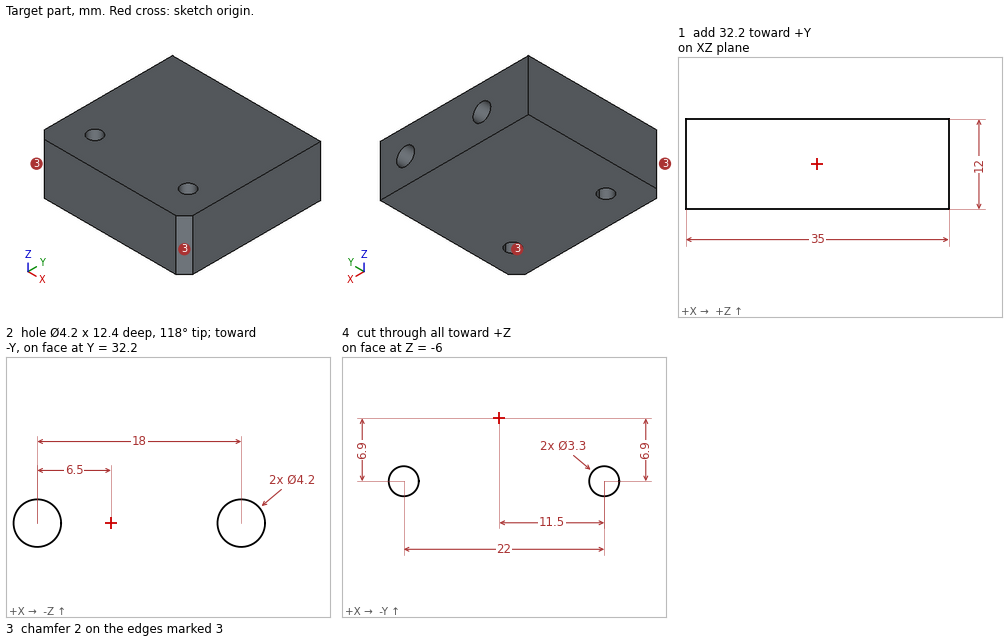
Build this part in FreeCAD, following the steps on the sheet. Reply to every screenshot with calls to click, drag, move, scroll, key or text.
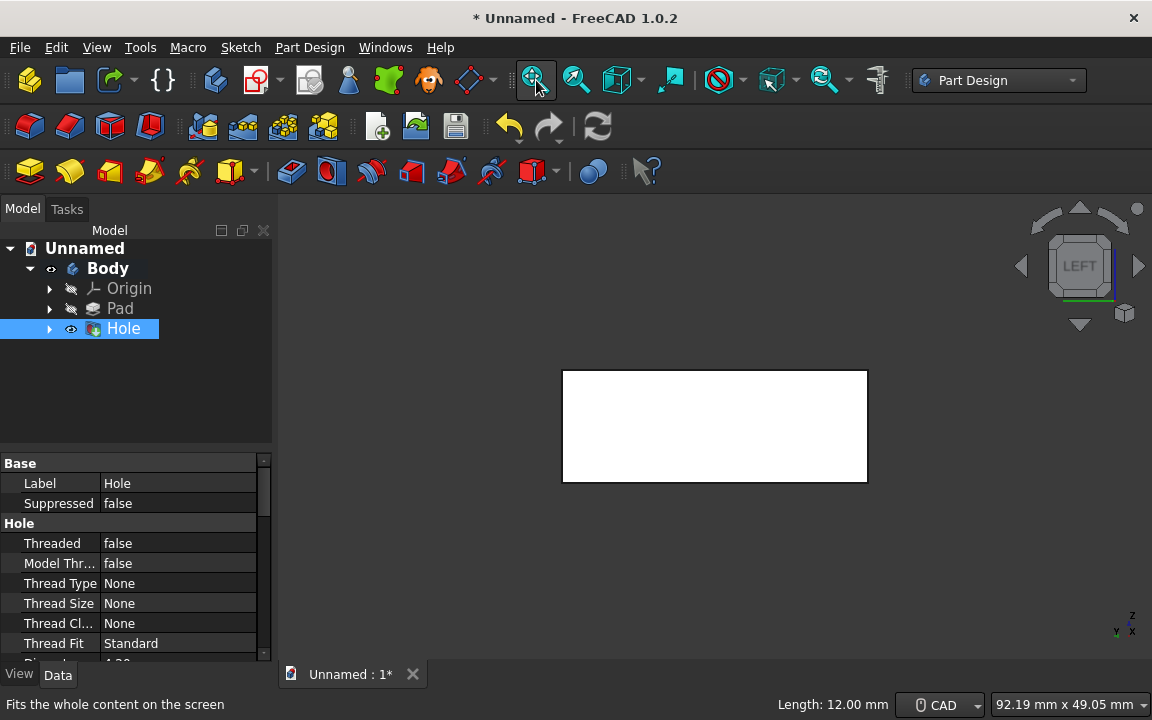
click(536, 80)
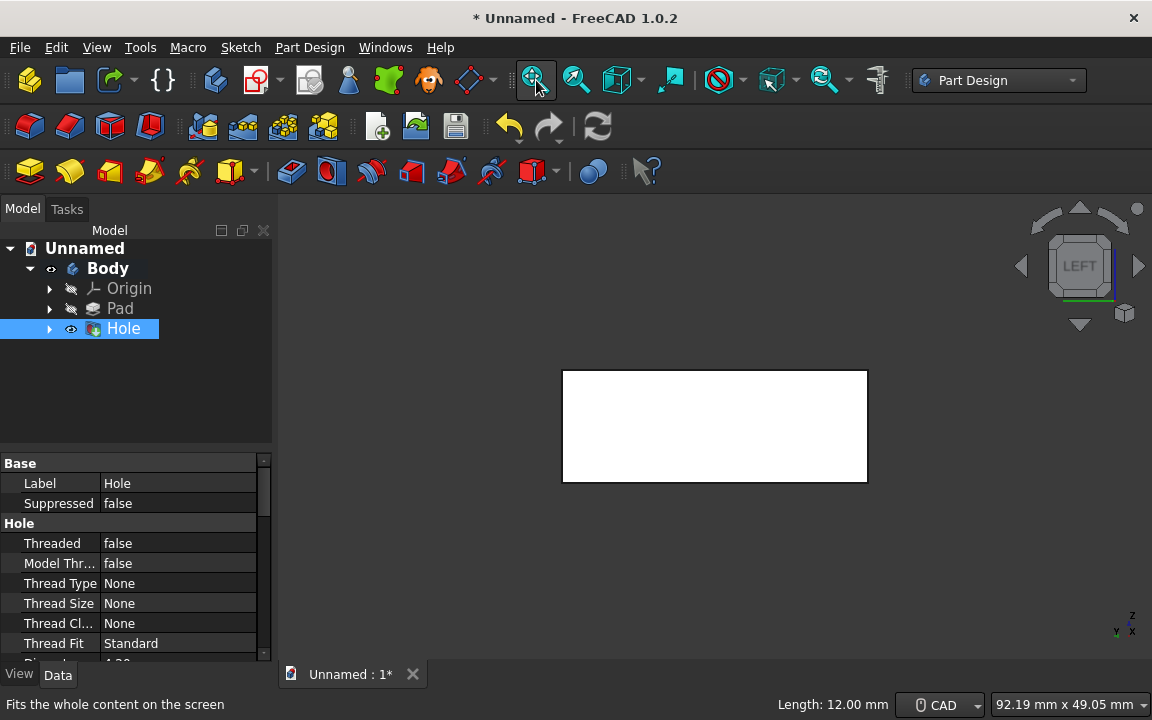
click(868, 426, ctrl)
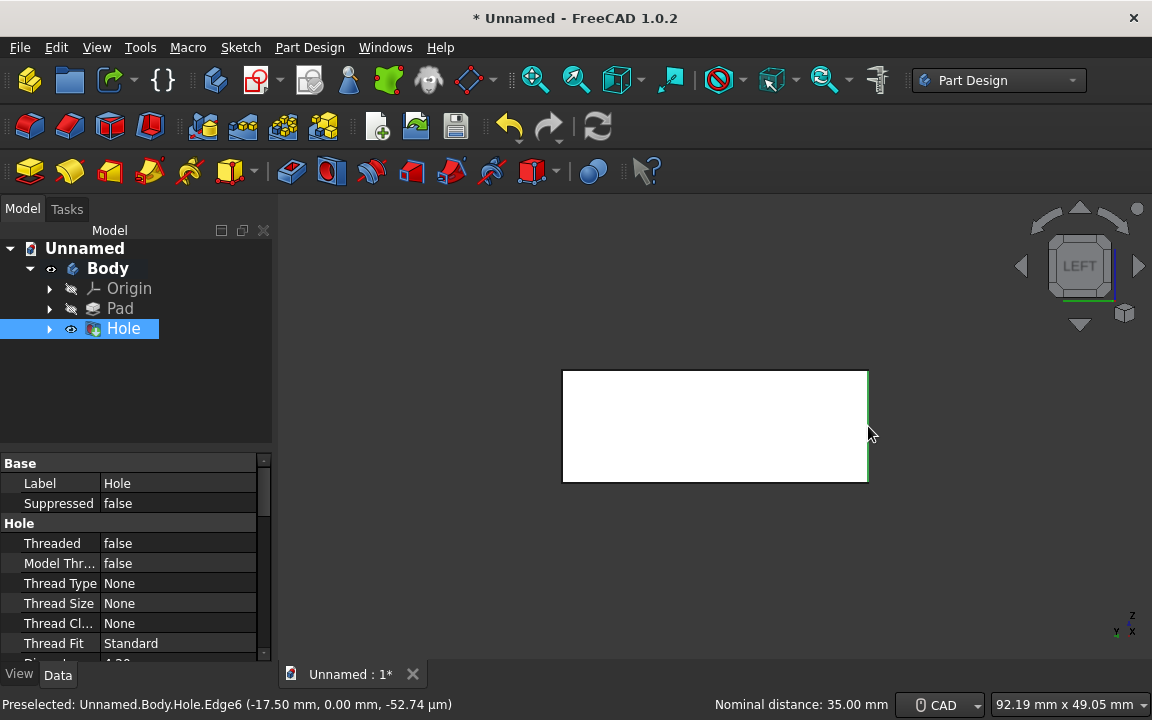
click(70, 126)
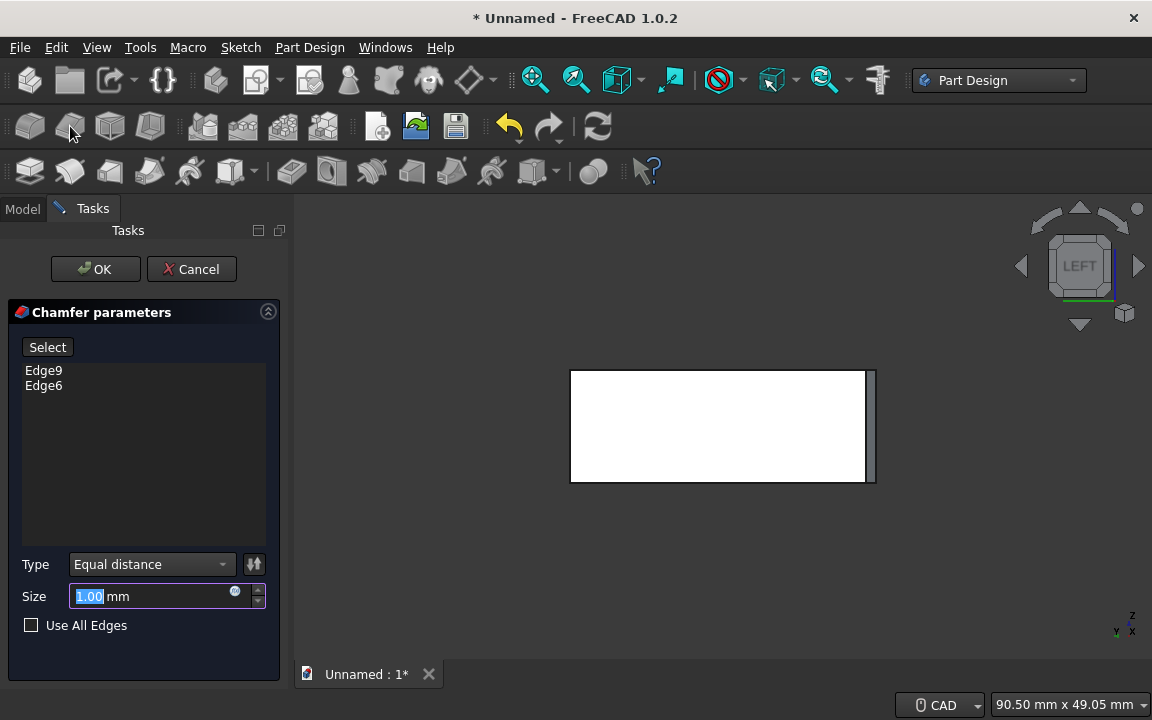
text(2)
key(Tab)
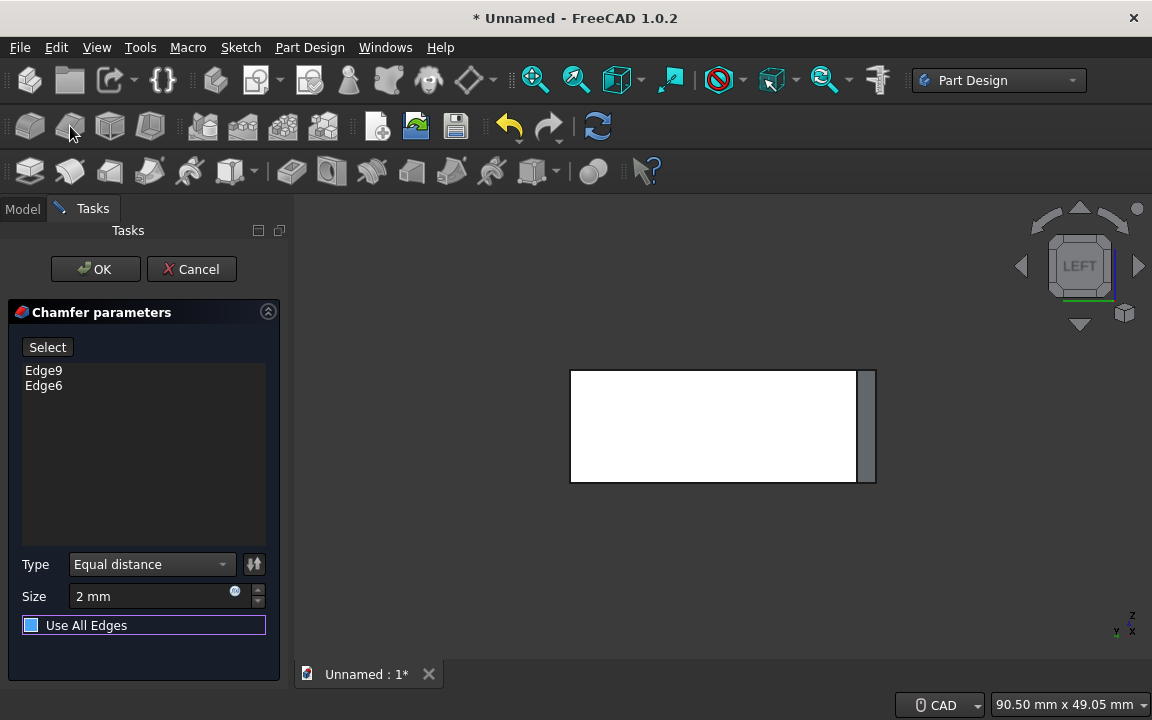
click(96, 269)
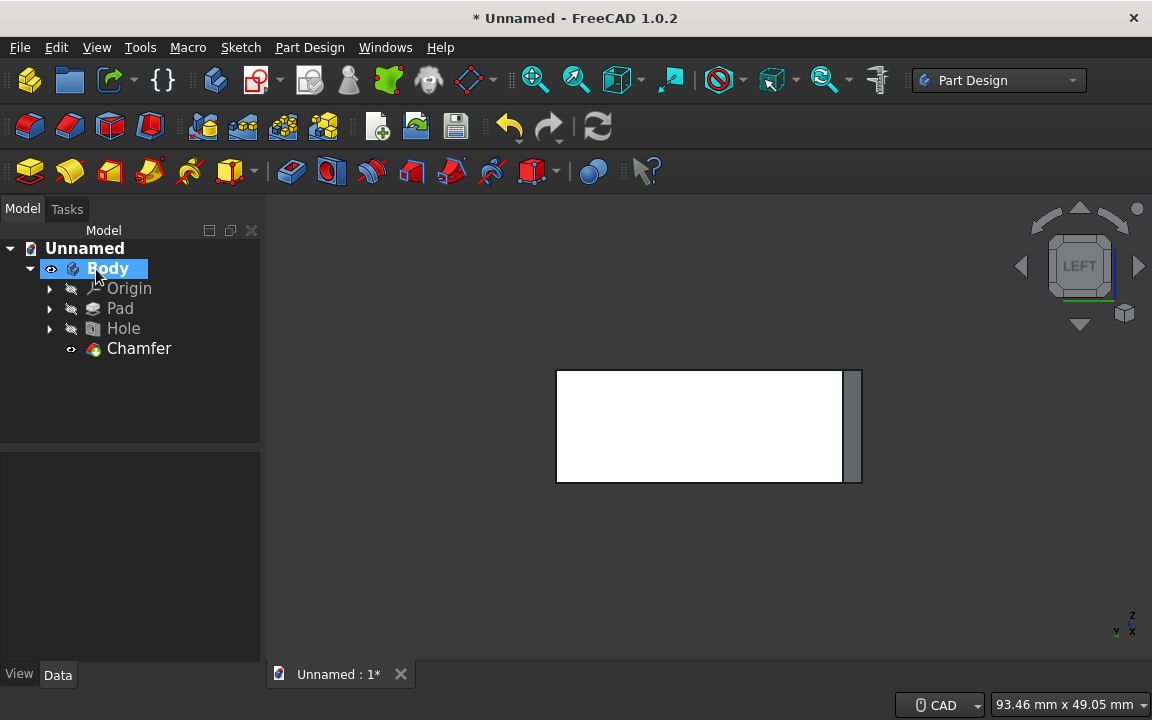
key(v)
key(f)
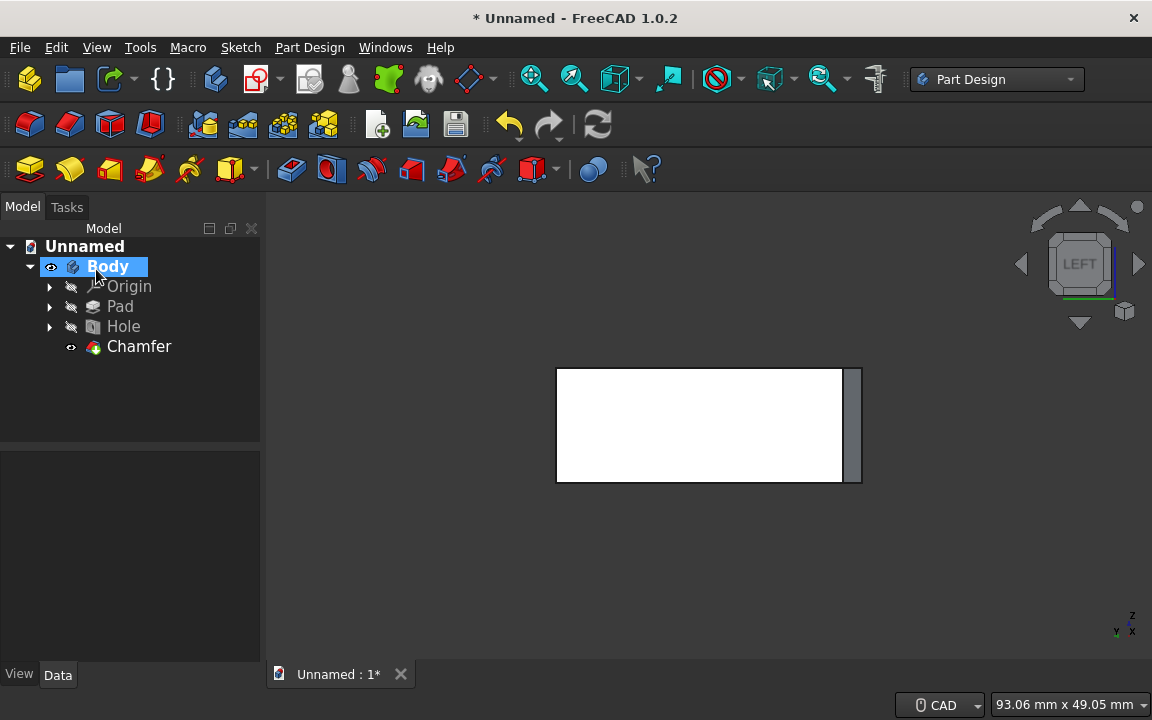
key(5)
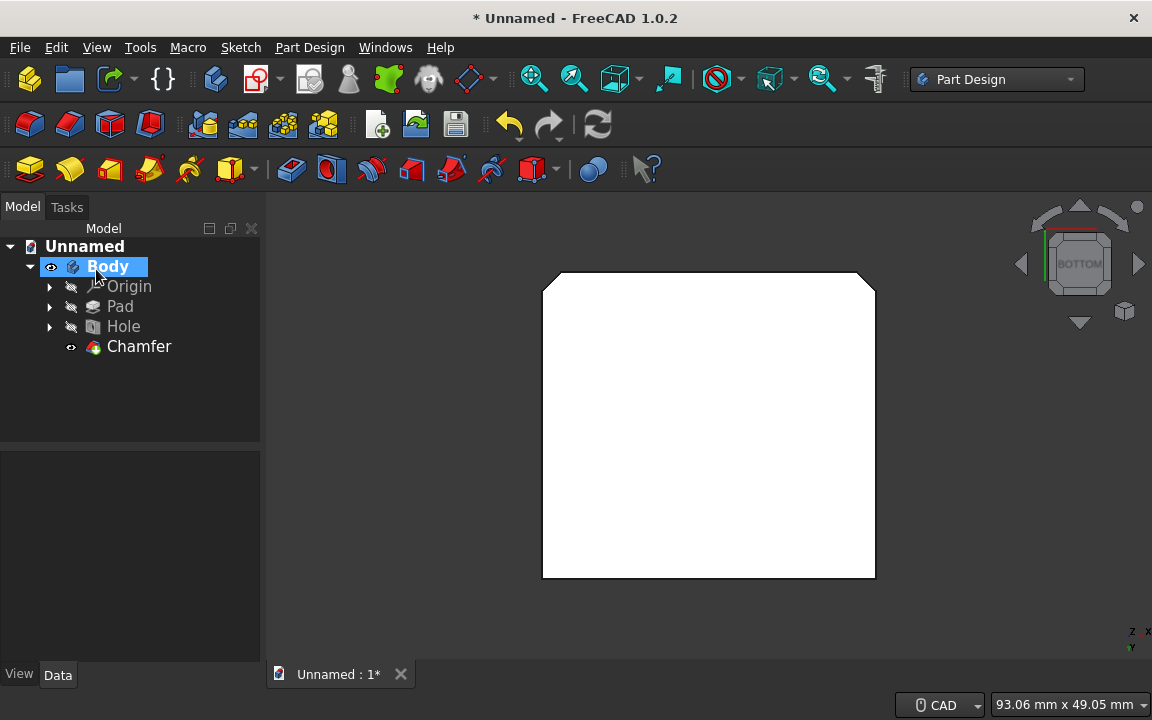
click(709, 424)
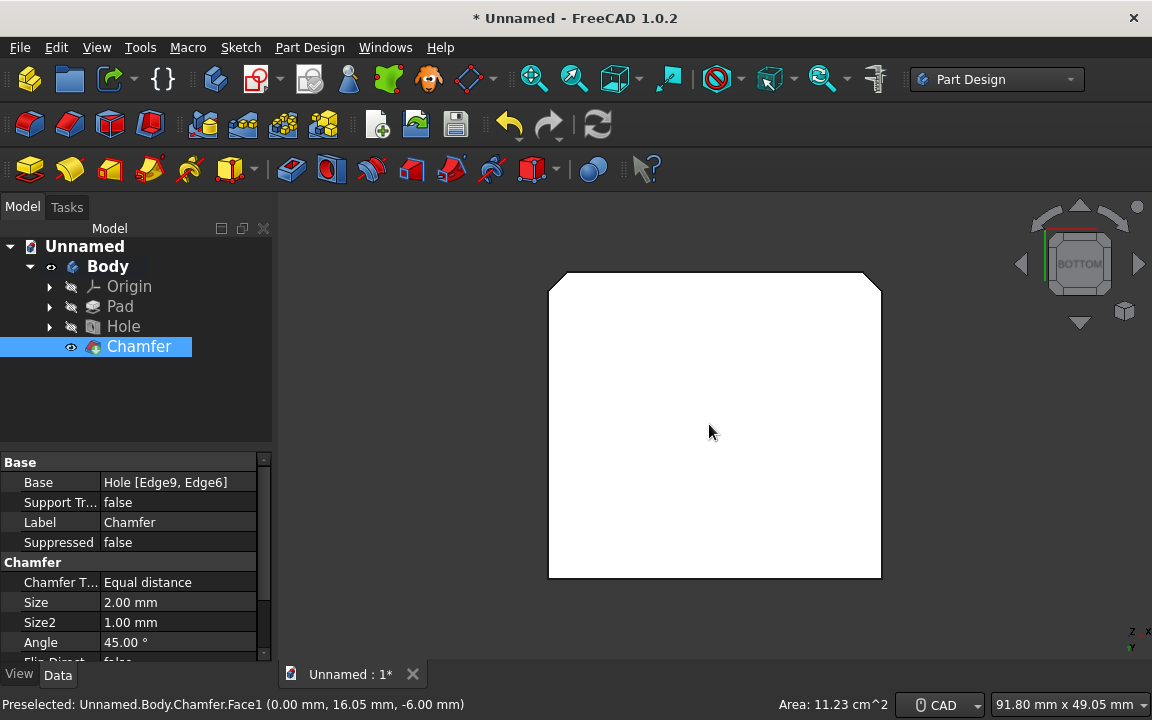
click(256, 80)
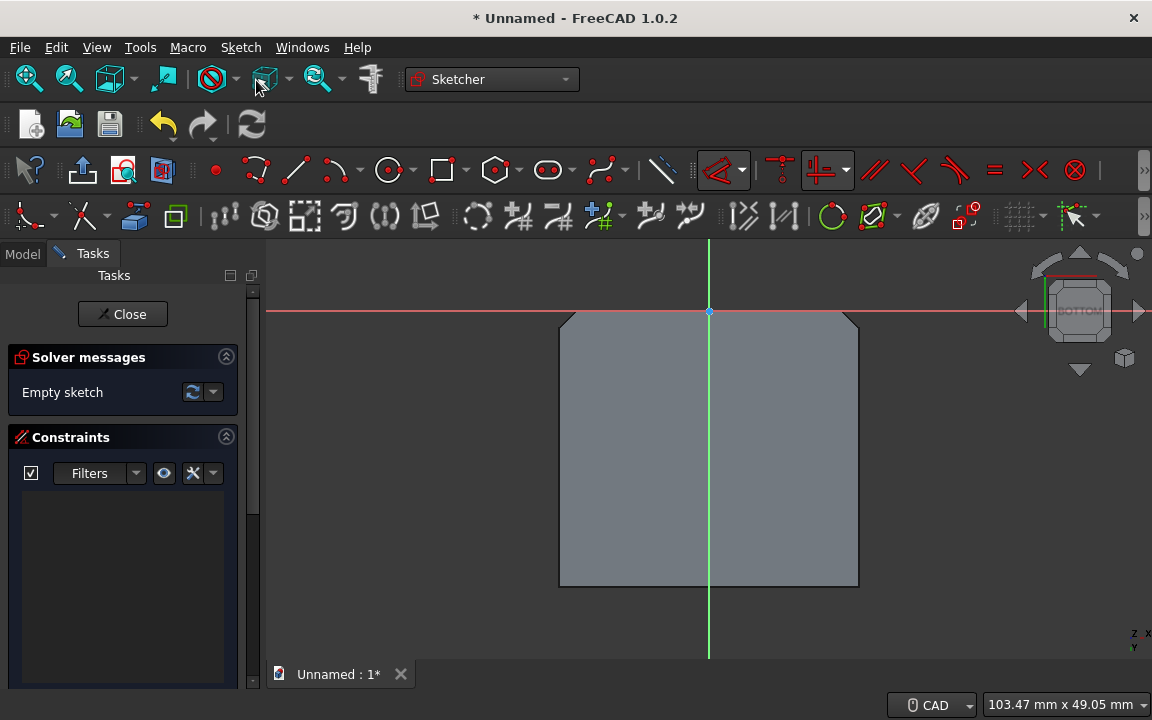
scroll(773, 267, up, 4)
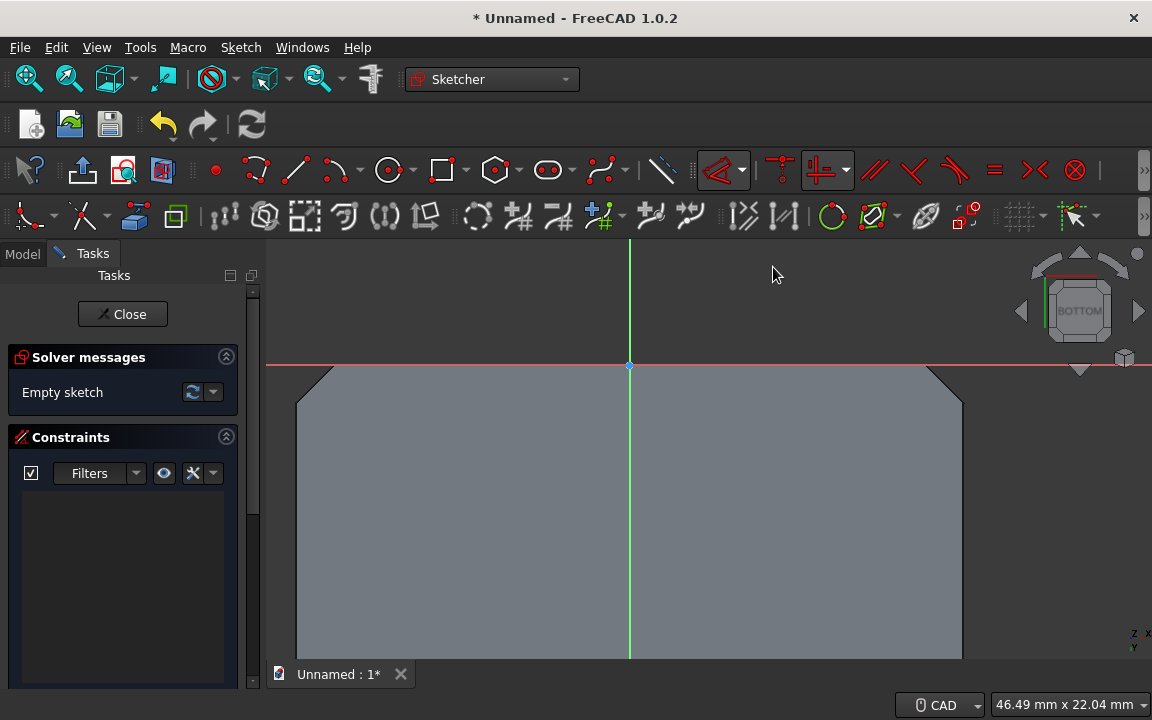
key(g)
key(c)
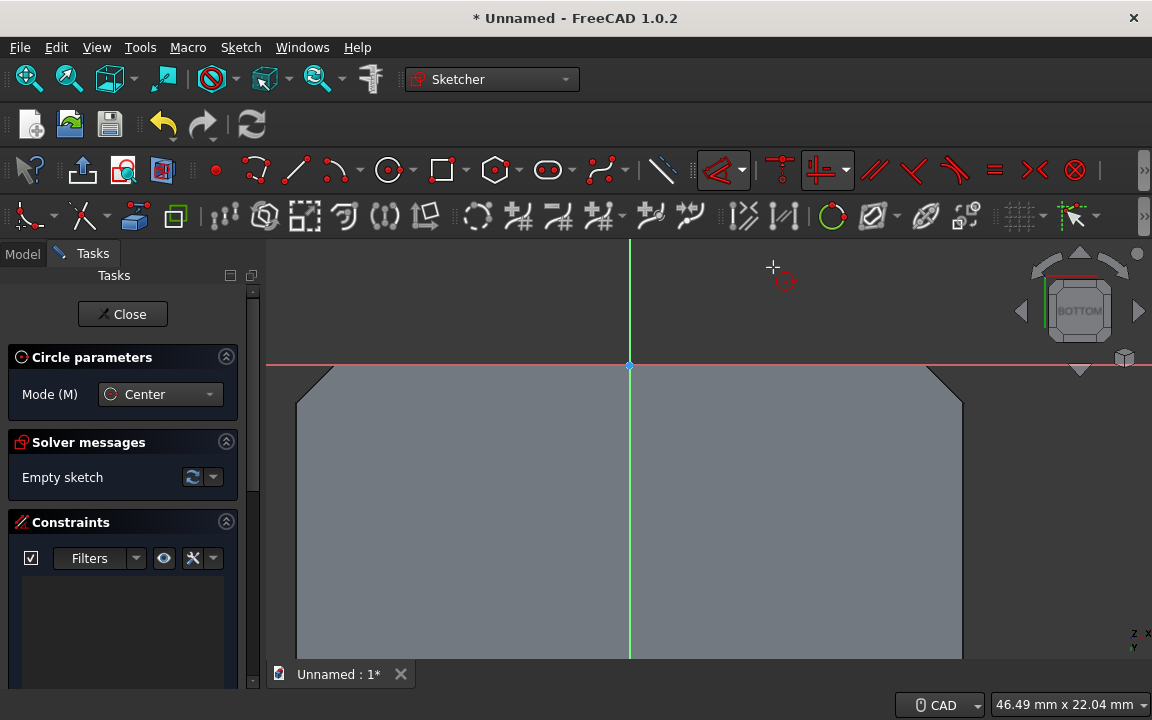
click(849, 497)
move(871, 474)